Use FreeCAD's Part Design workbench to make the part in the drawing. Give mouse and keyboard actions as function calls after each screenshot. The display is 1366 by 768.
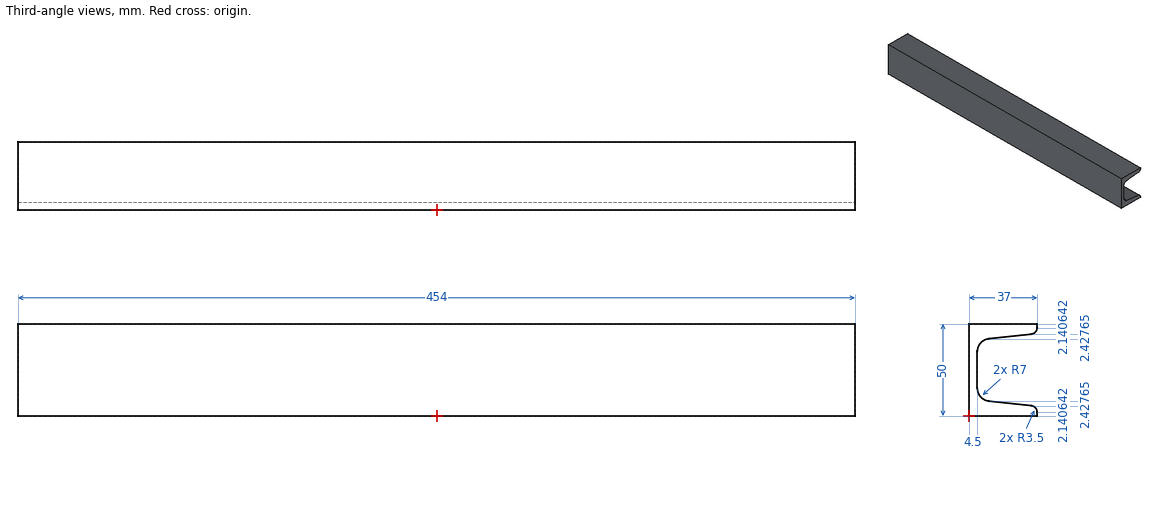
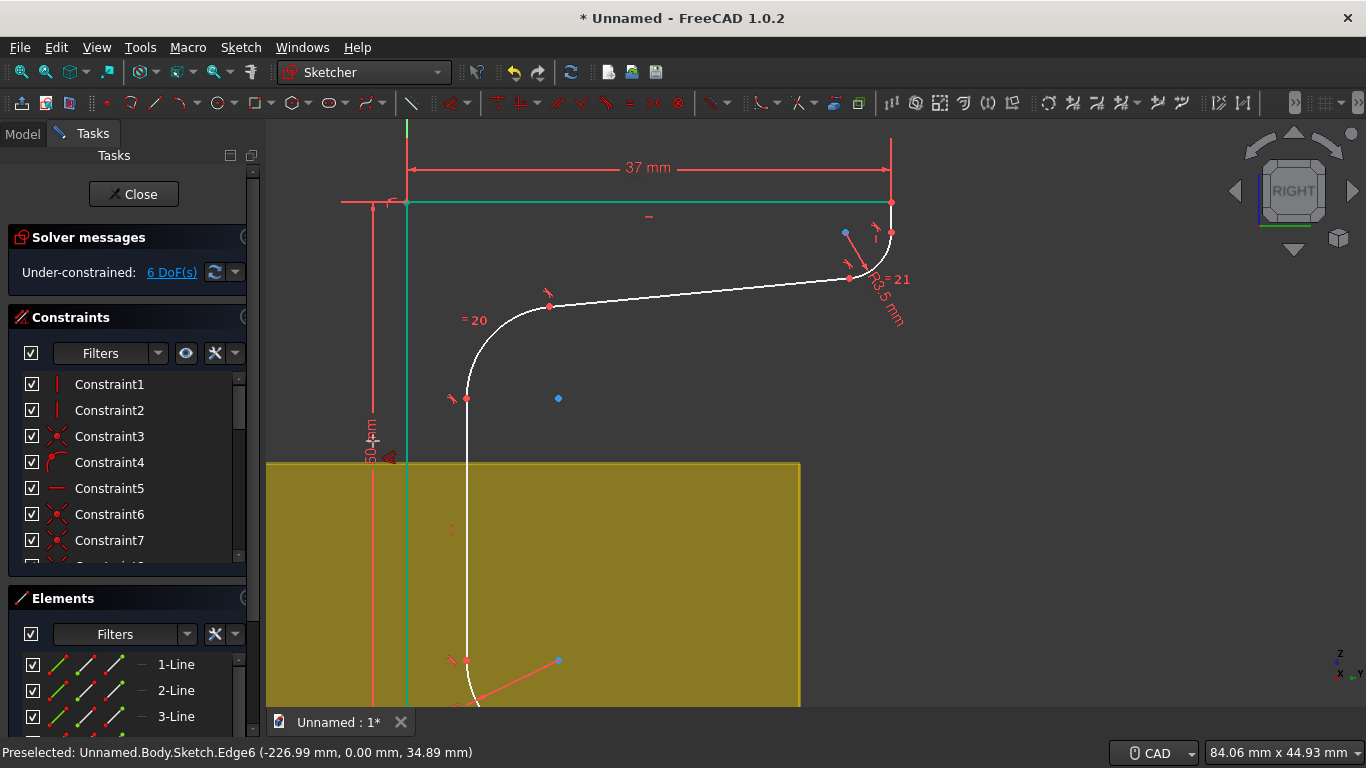
scroll(867, 271, down, 3)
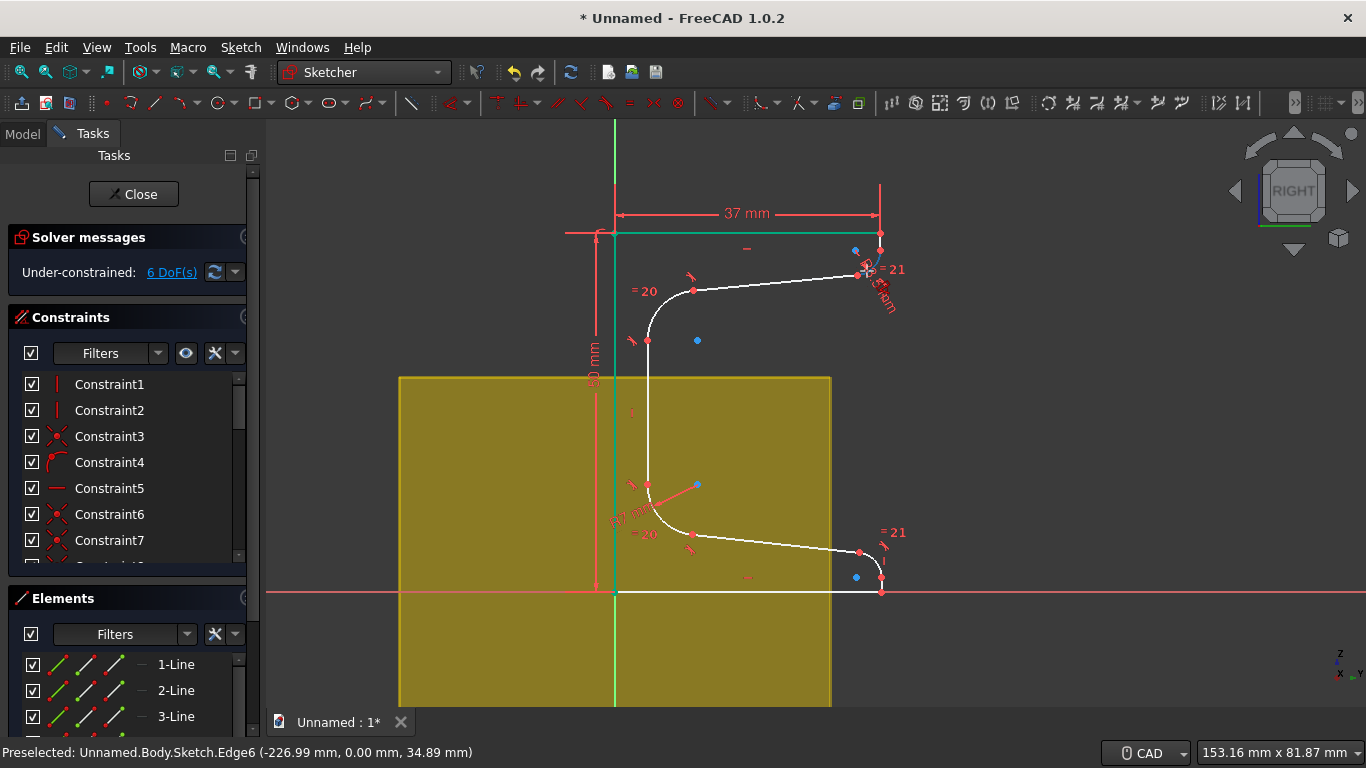
click(695, 592)
click(748, 626)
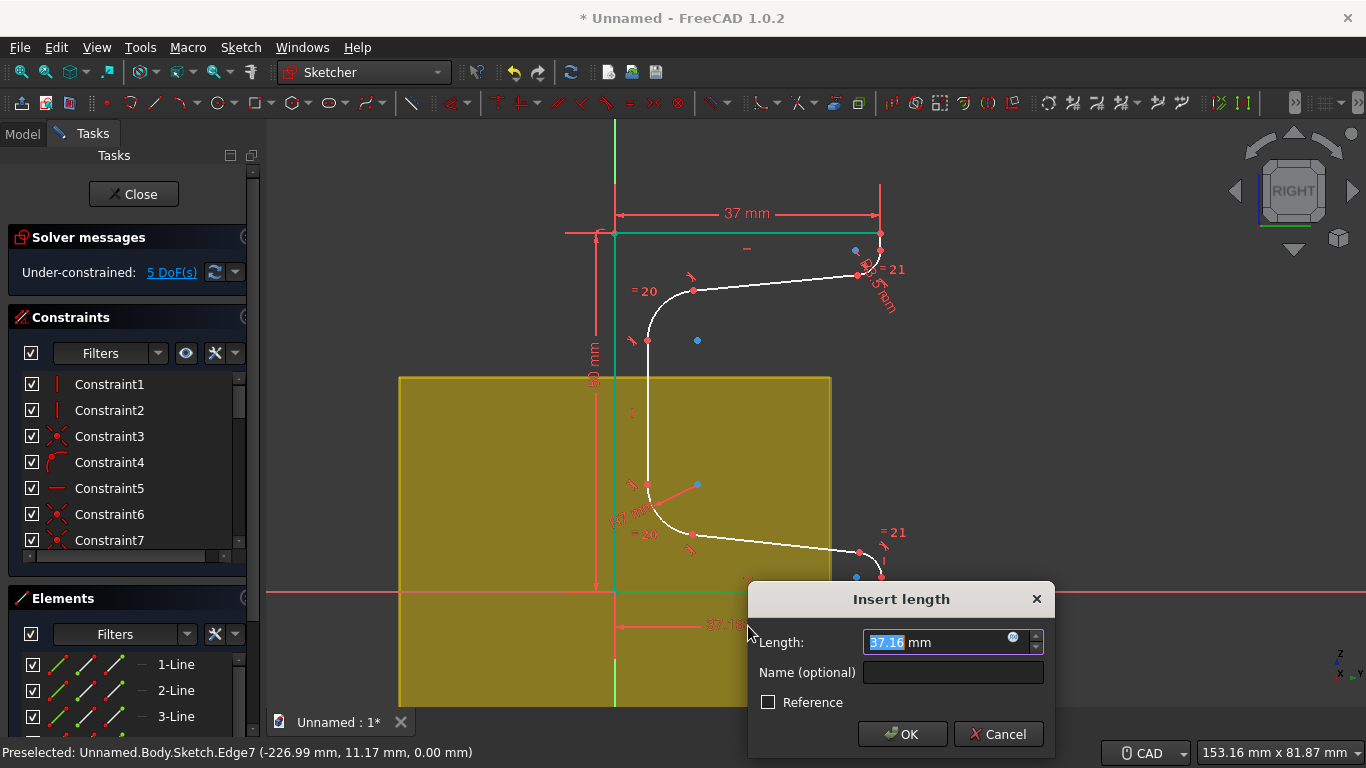
text(37)
key(Return)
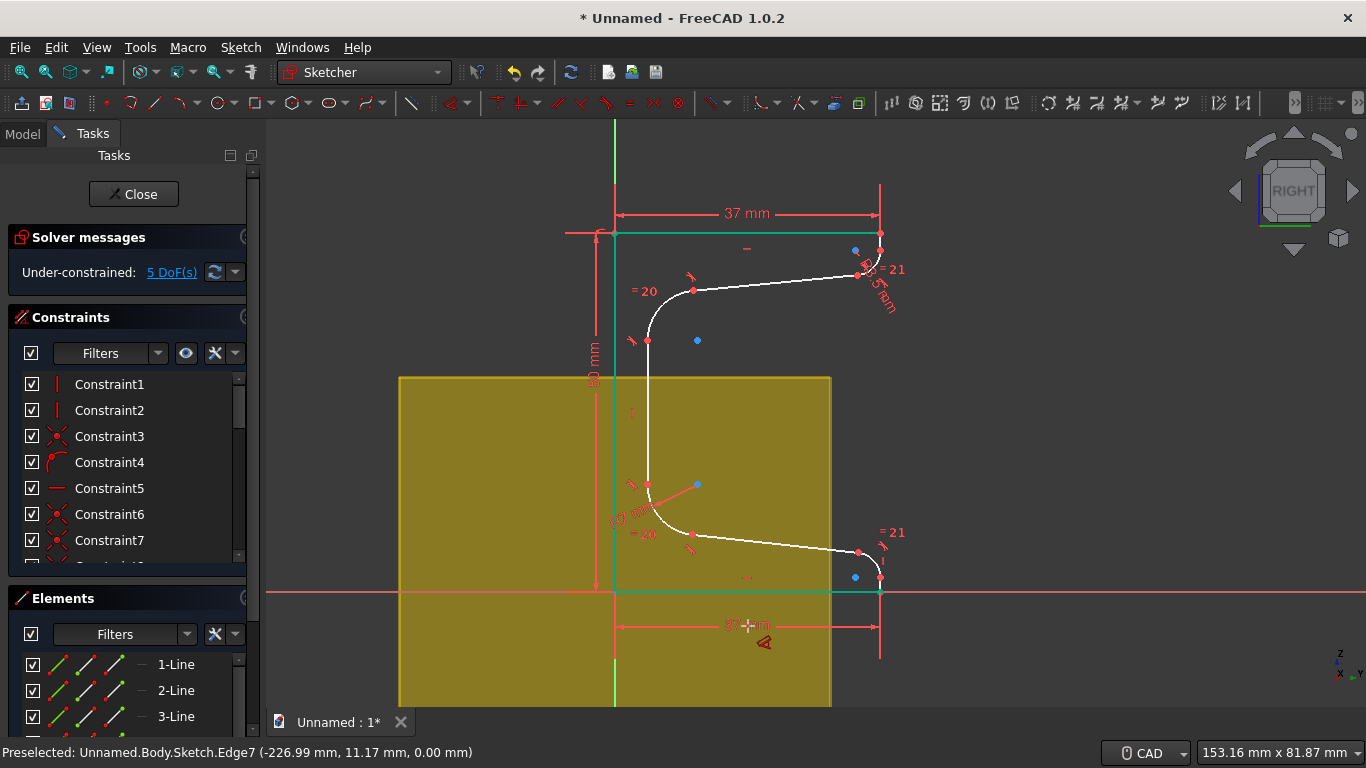
scroll(648, 485, up, 2)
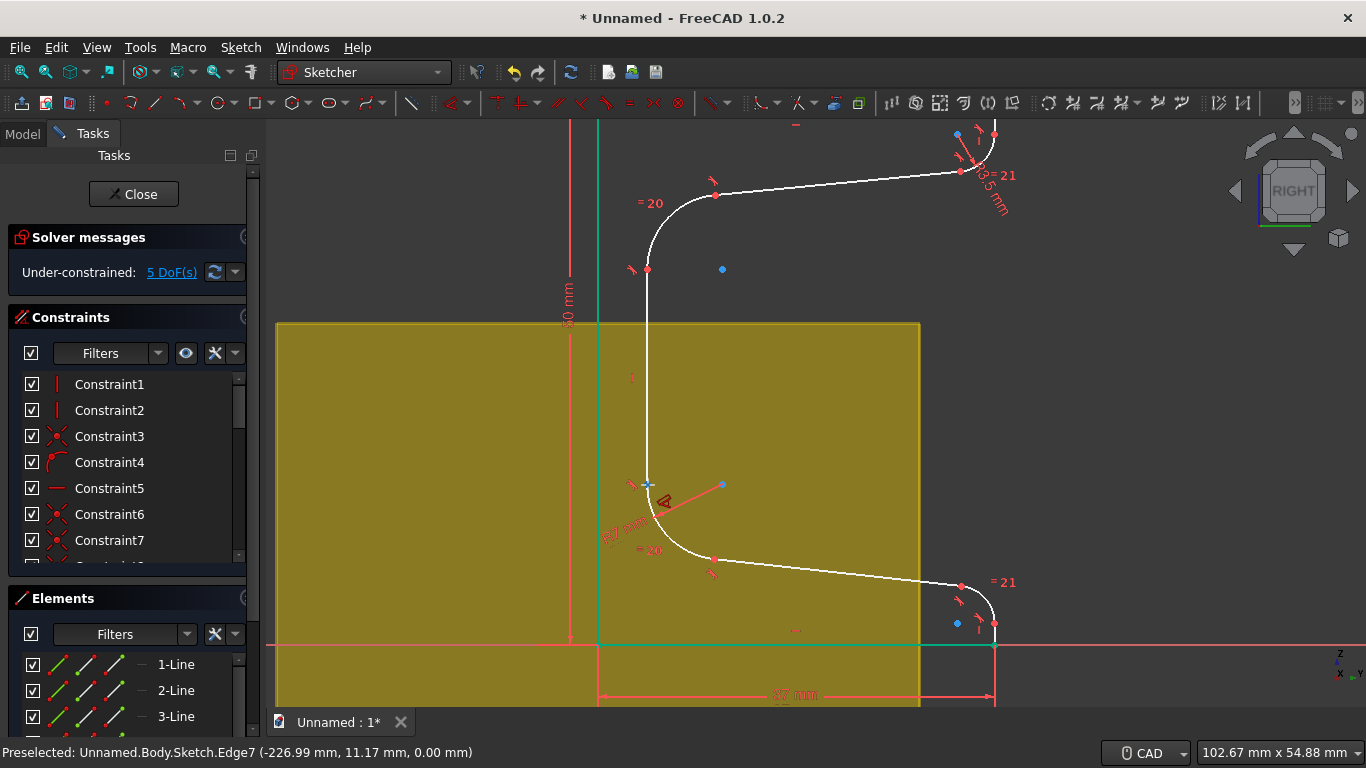
click(647, 485)
click(623, 451)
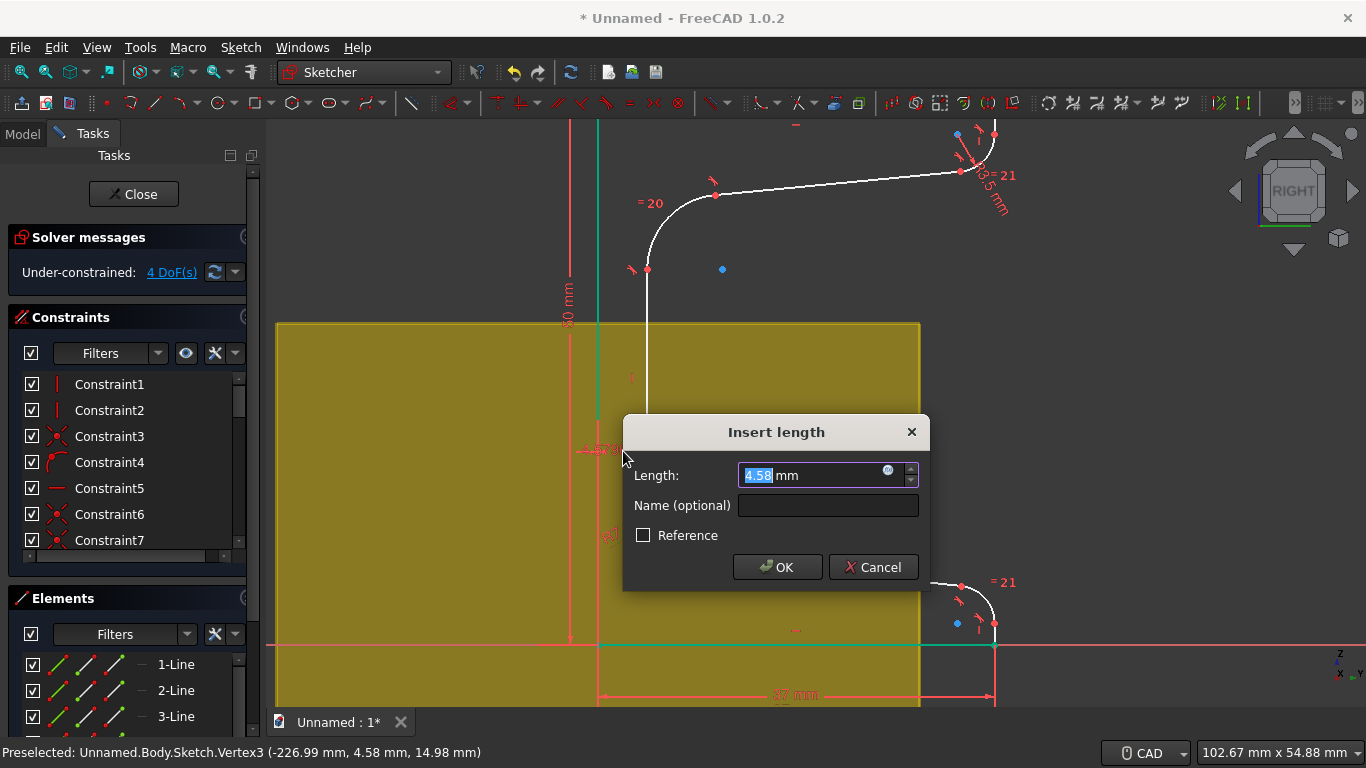
text(4.5)
key(Return)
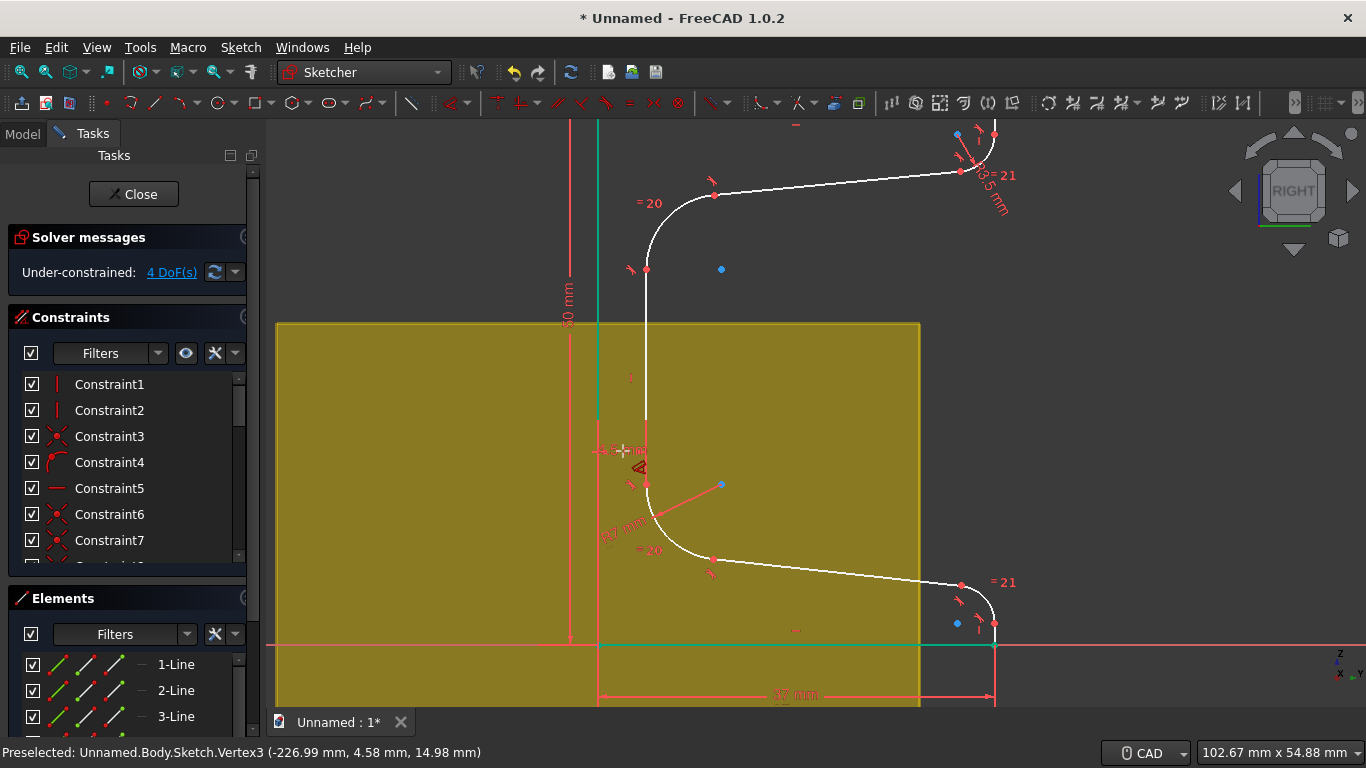
scroll(648, 486, down, 2)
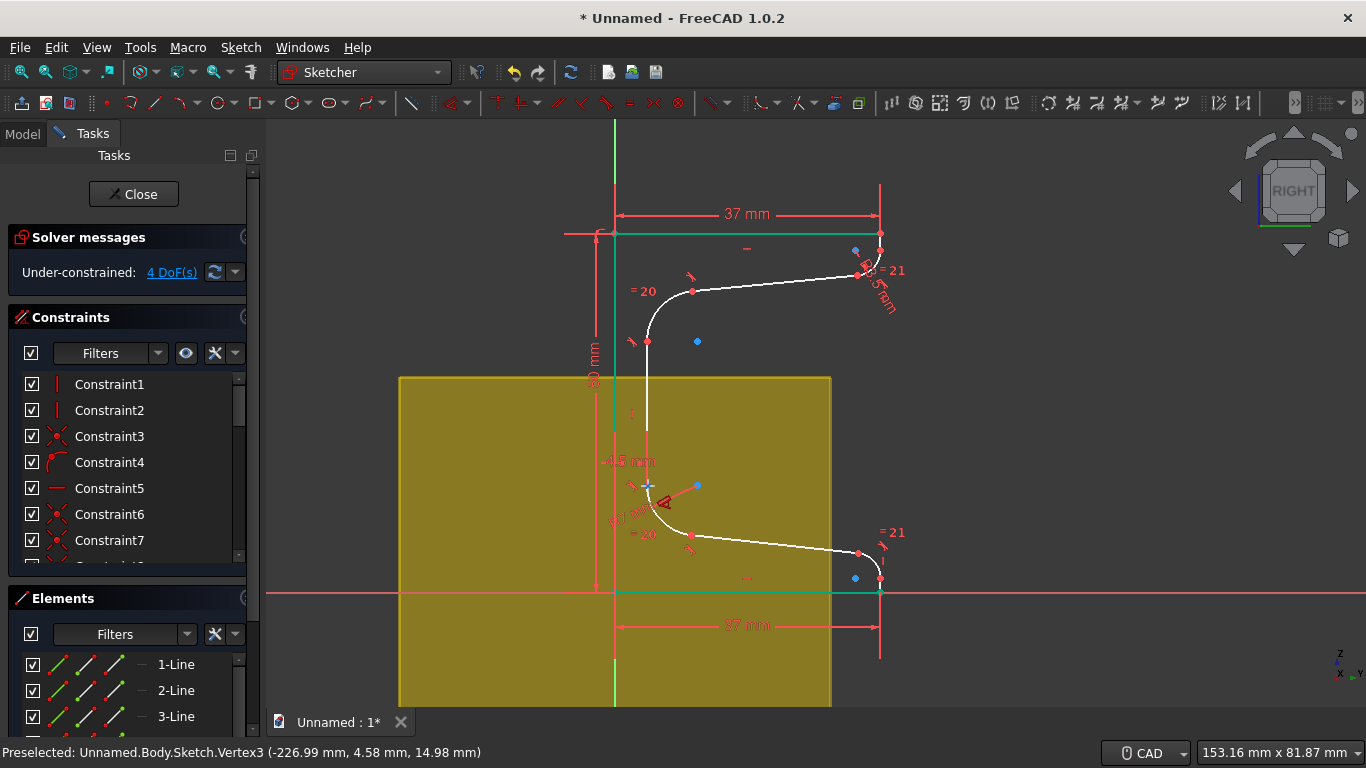
scroll(880, 244, up, 5)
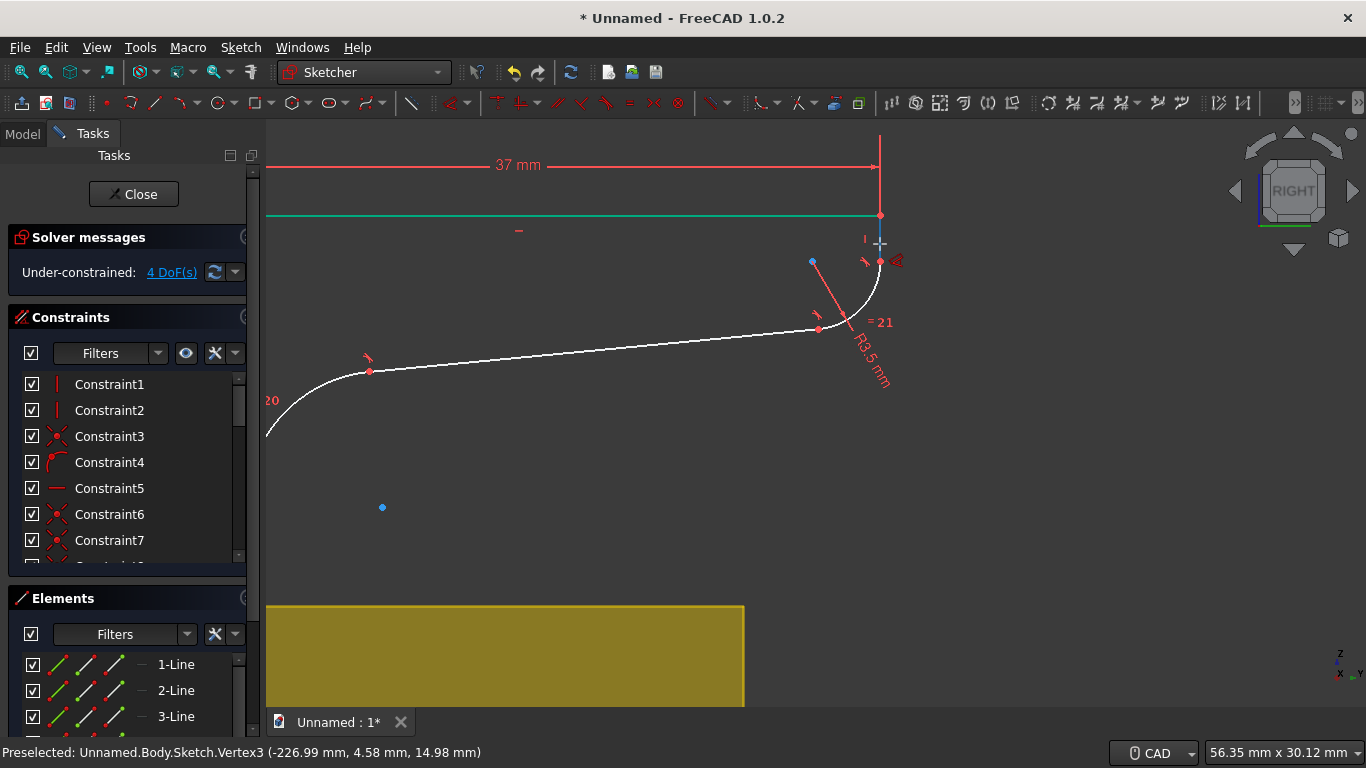
click(880, 243)
click(914, 238)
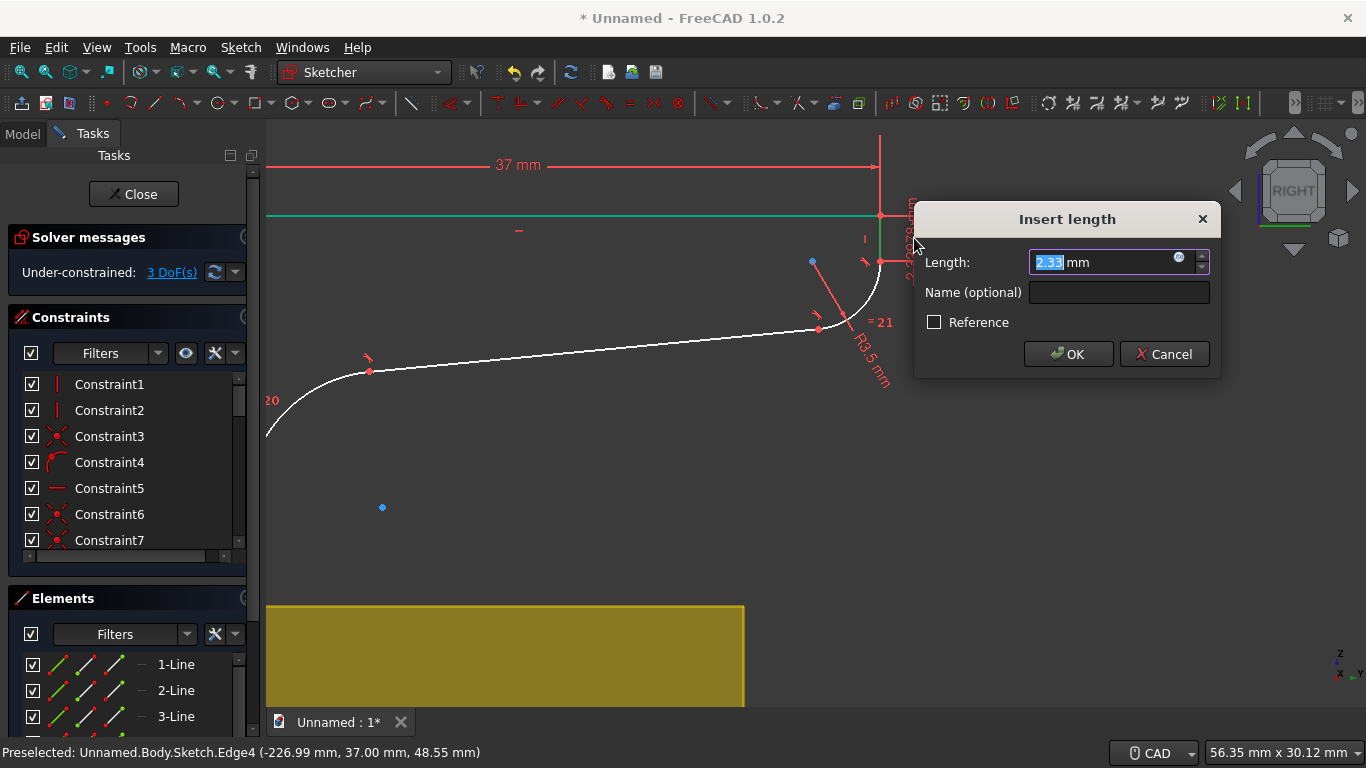
text(2.140642)
key(Return)